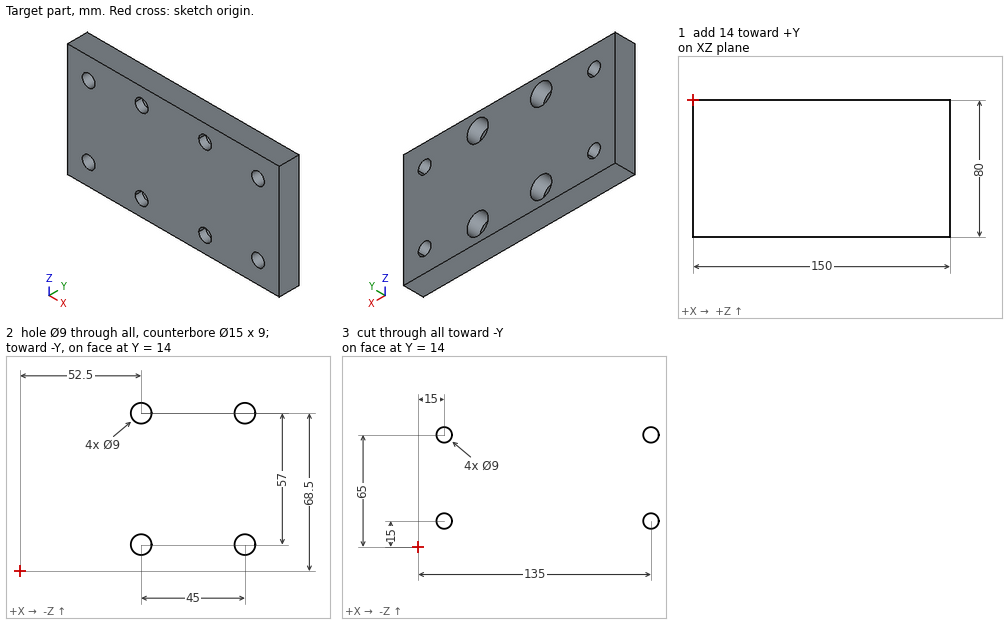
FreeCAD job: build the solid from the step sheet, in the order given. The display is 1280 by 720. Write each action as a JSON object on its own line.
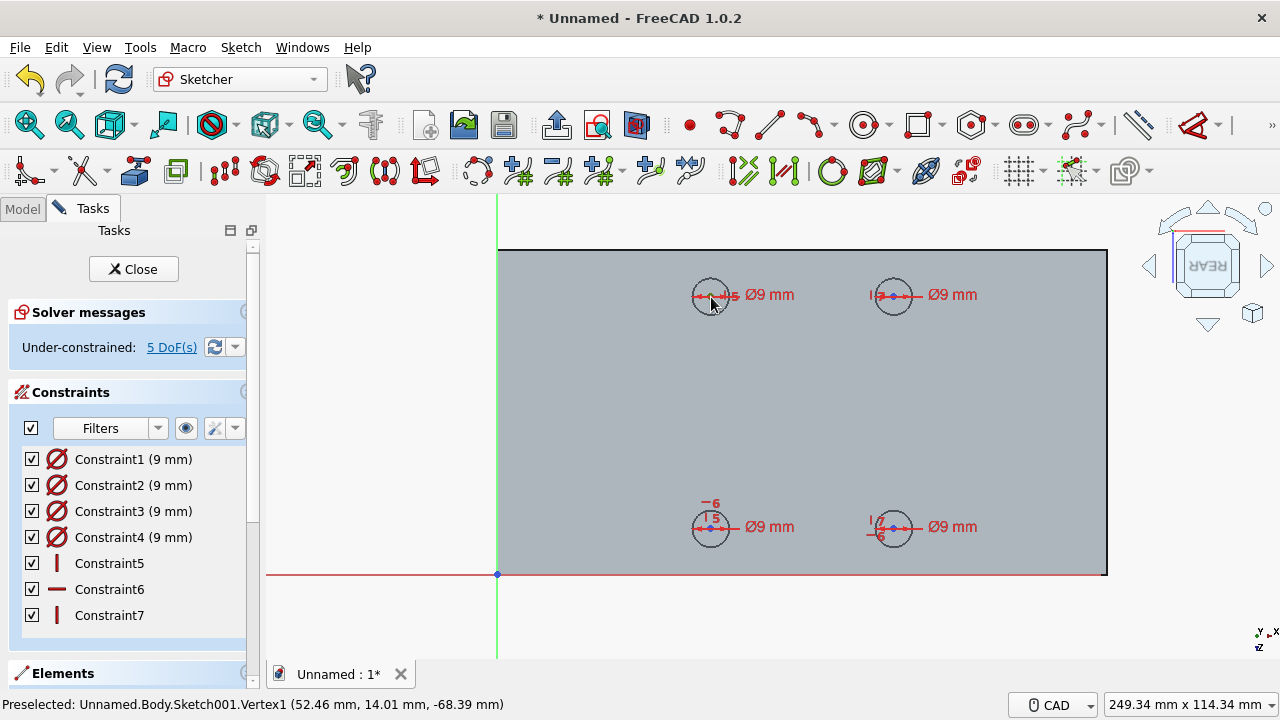
{"action": "left_click", "coordinate": [894, 297]}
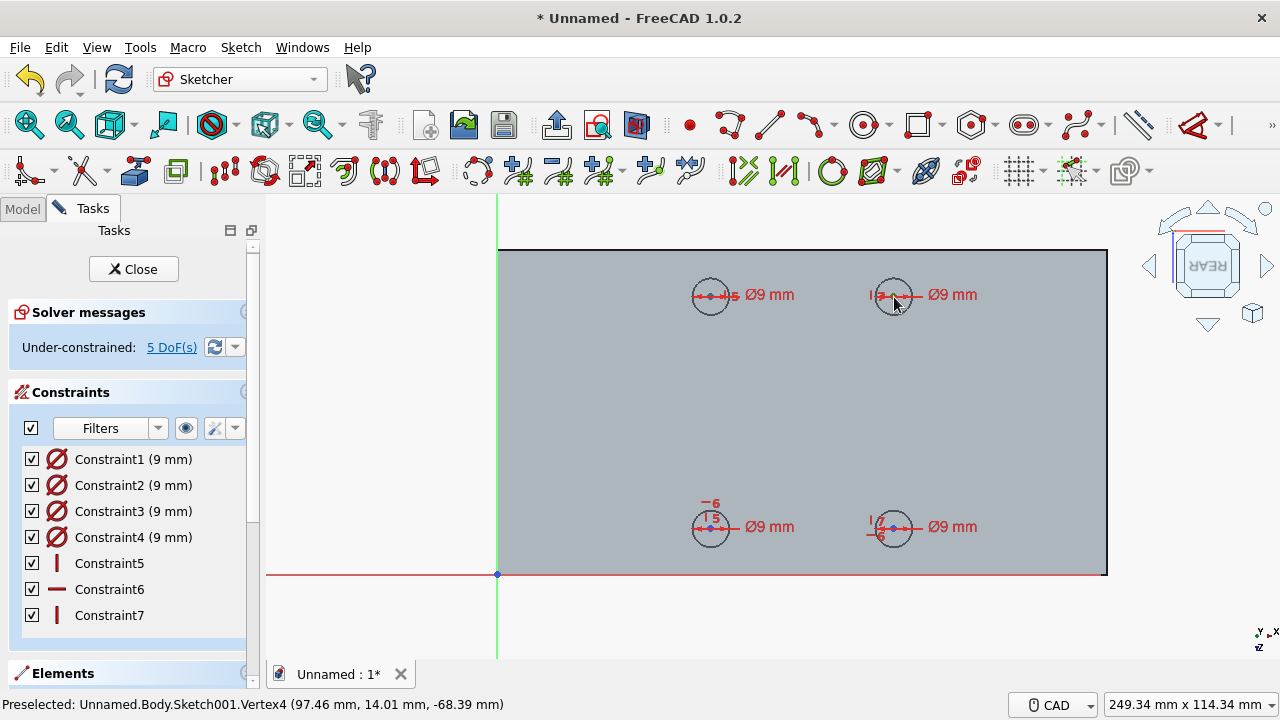
{"action": "key", "text": "h"}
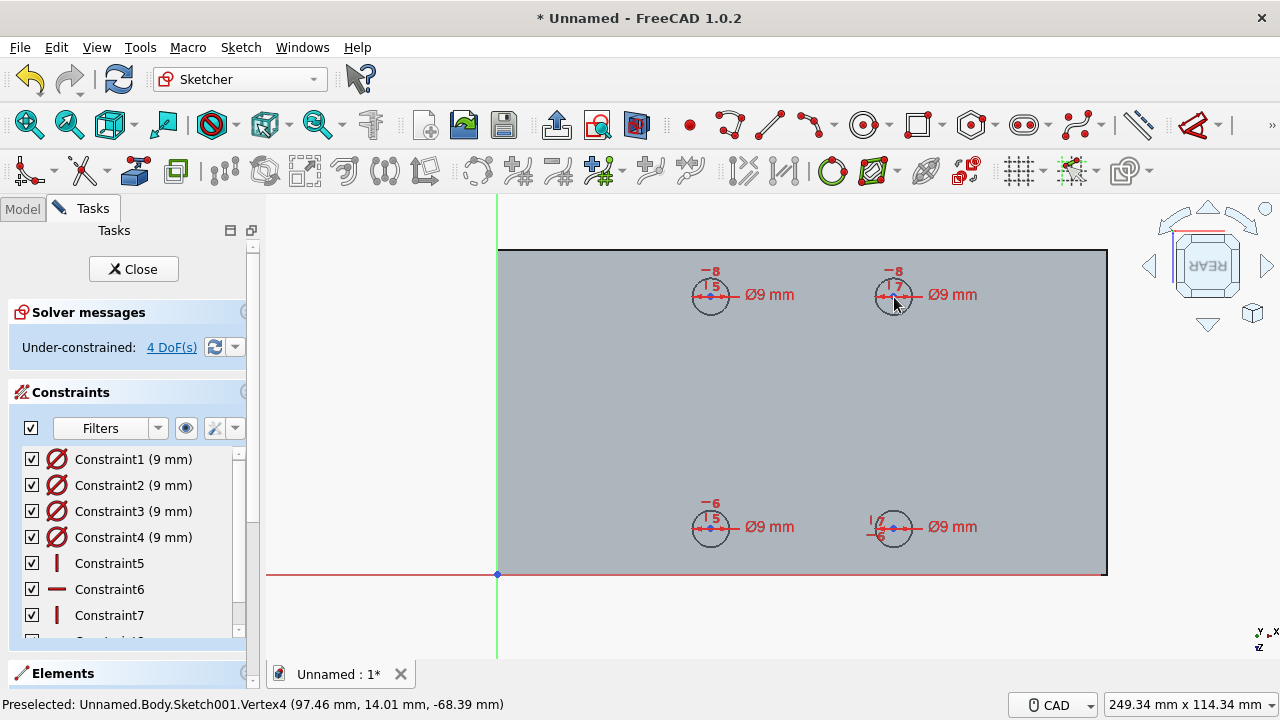
{"action": "left_click", "coordinate": [711, 297]}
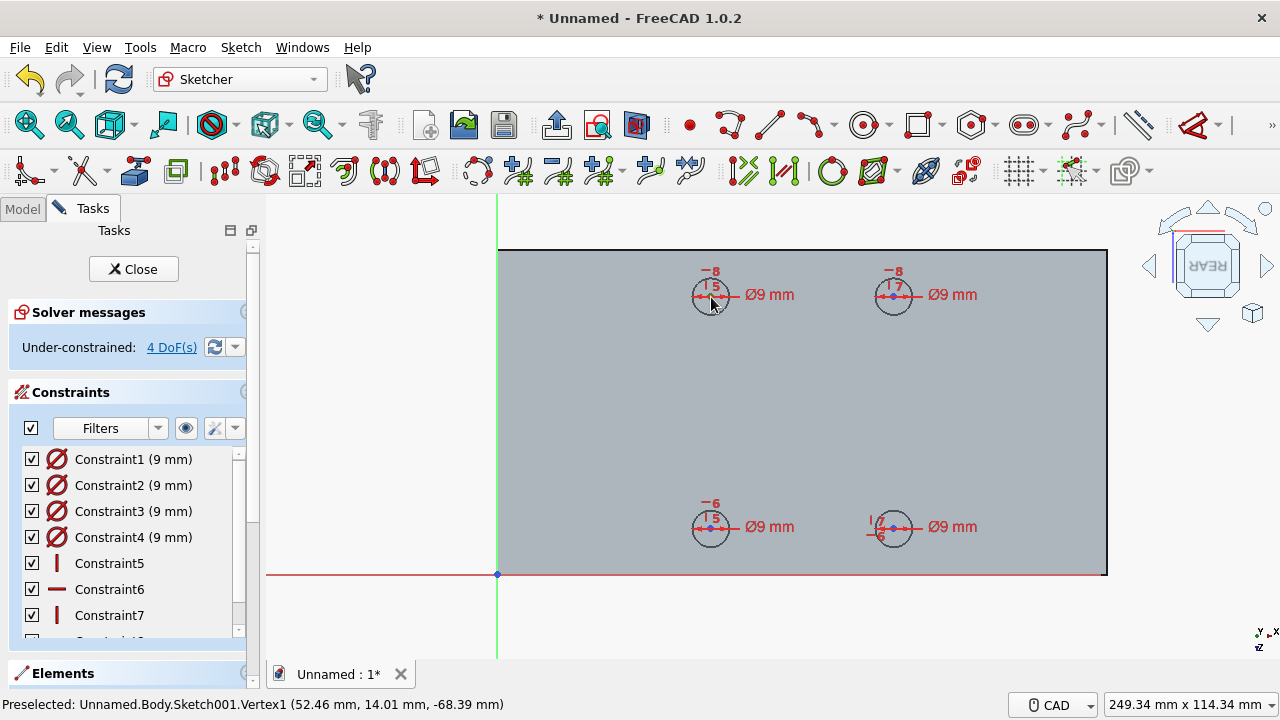
{"action": "left_click", "coordinate": [711, 529]}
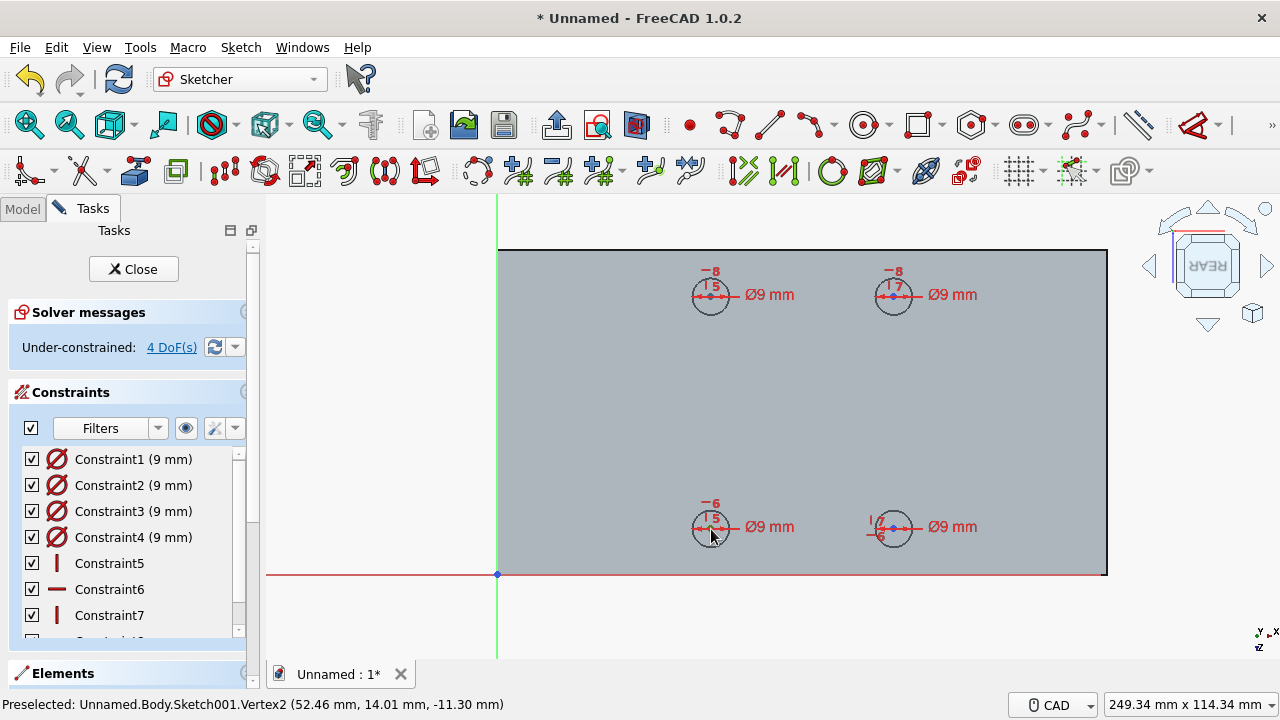
{"action": "left_click", "coordinate": [1220, 126]}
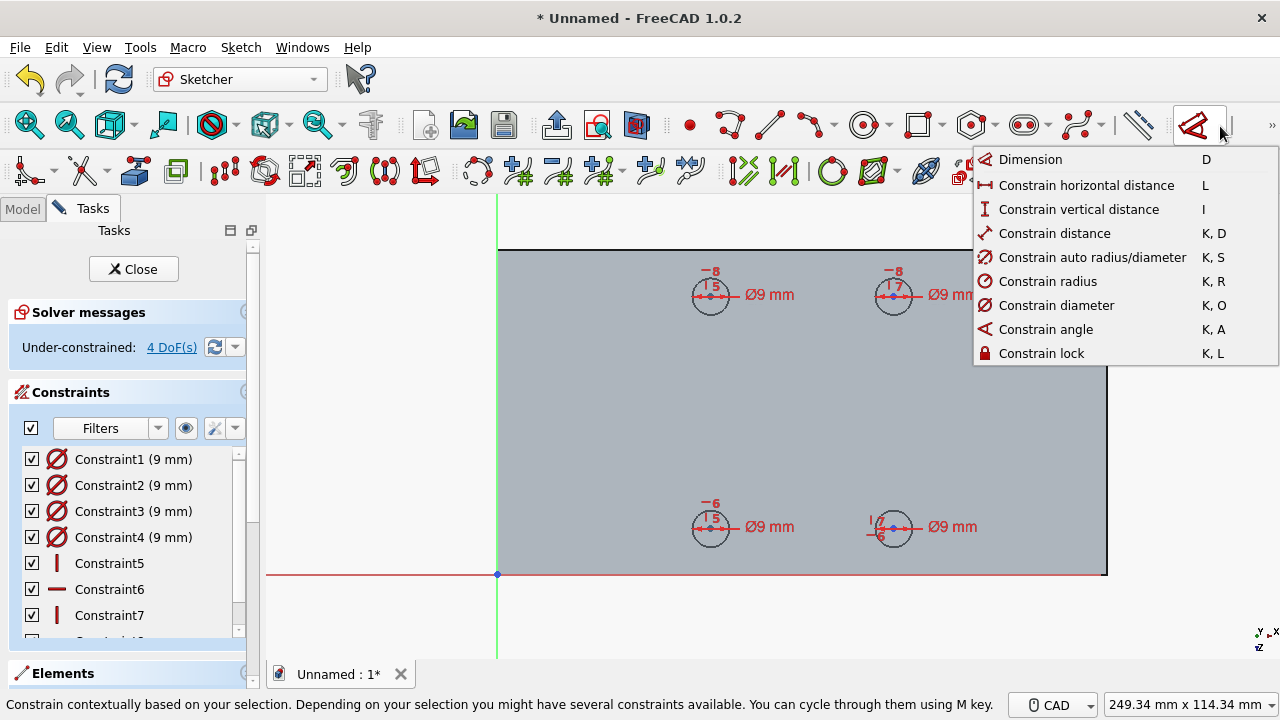
{"action": "left_click", "coordinate": [1126, 209]}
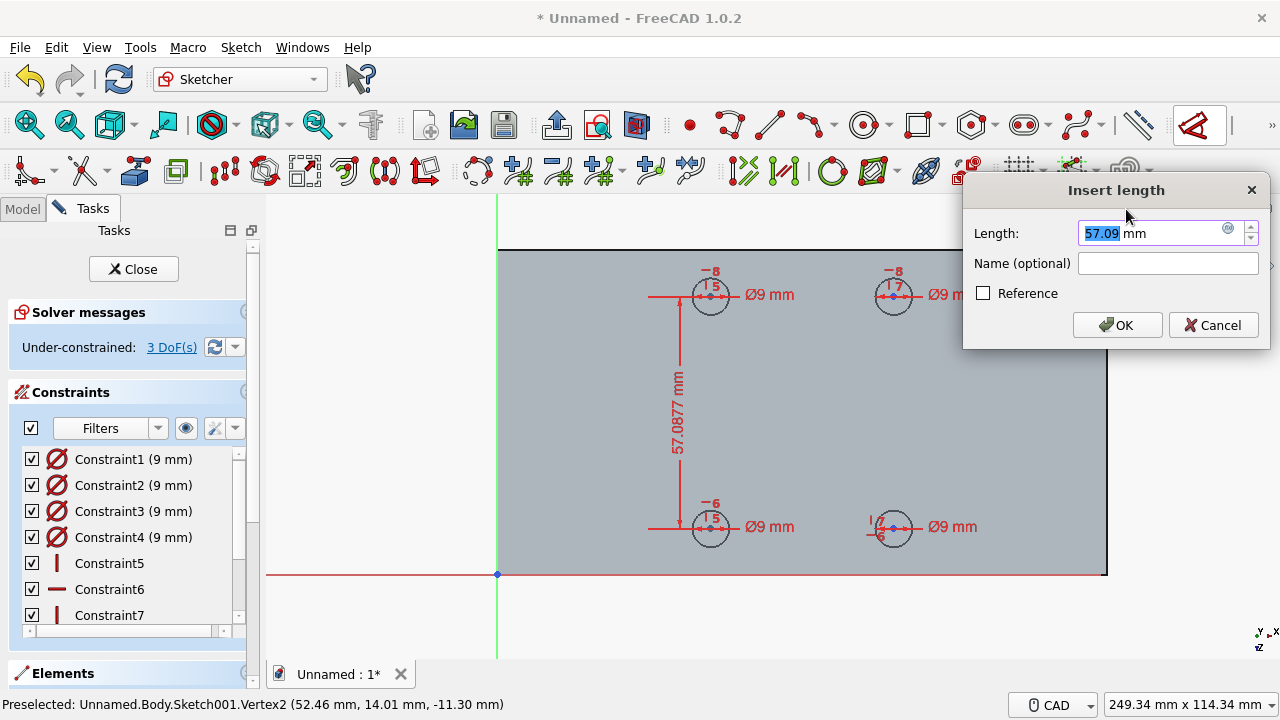
{"action": "type", "text": "57"}
{"action": "key", "text": "Return"}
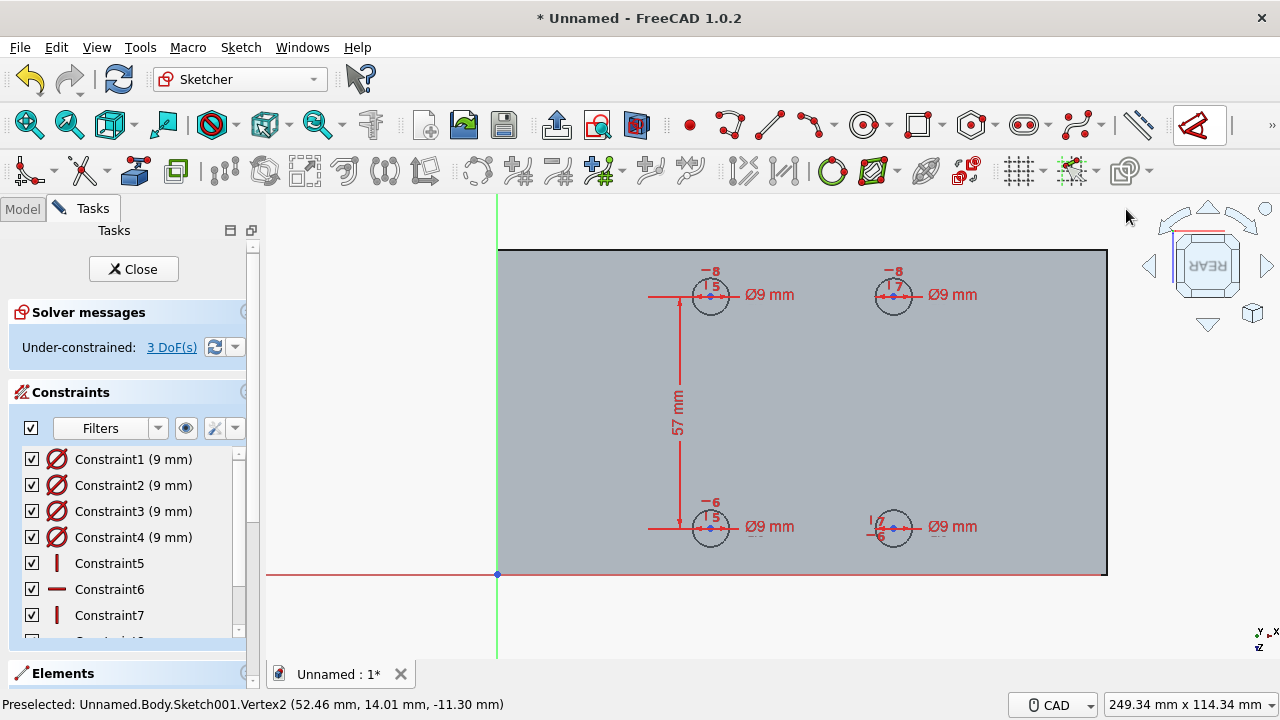
{"action": "left_click", "coordinate": [711, 529]}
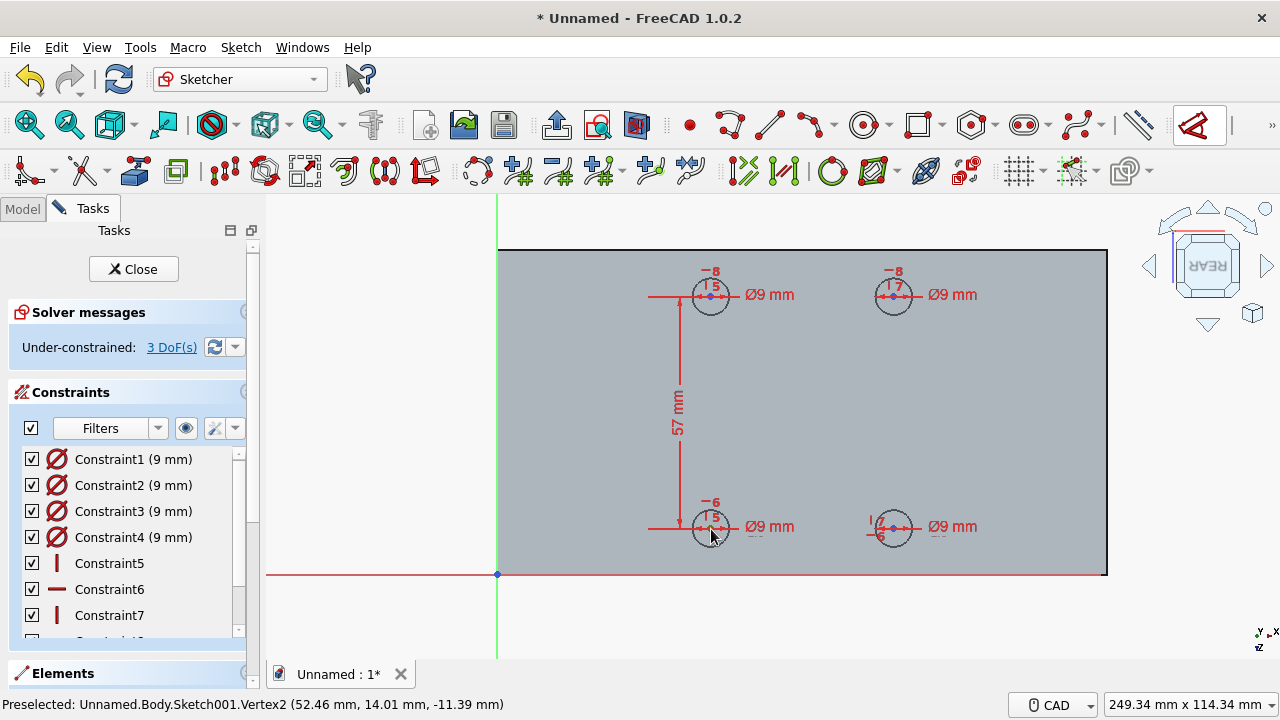
{"action": "left_click", "coordinate": [894, 529]}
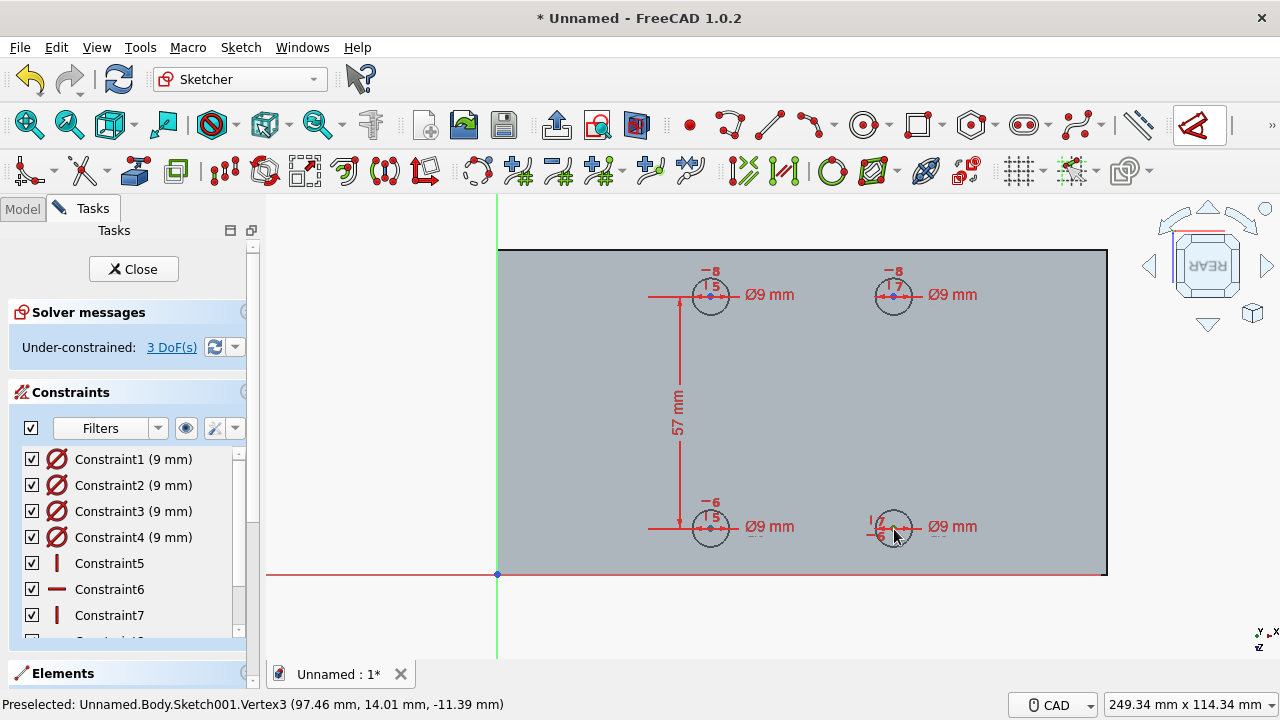
{"action": "key", "text": "l"}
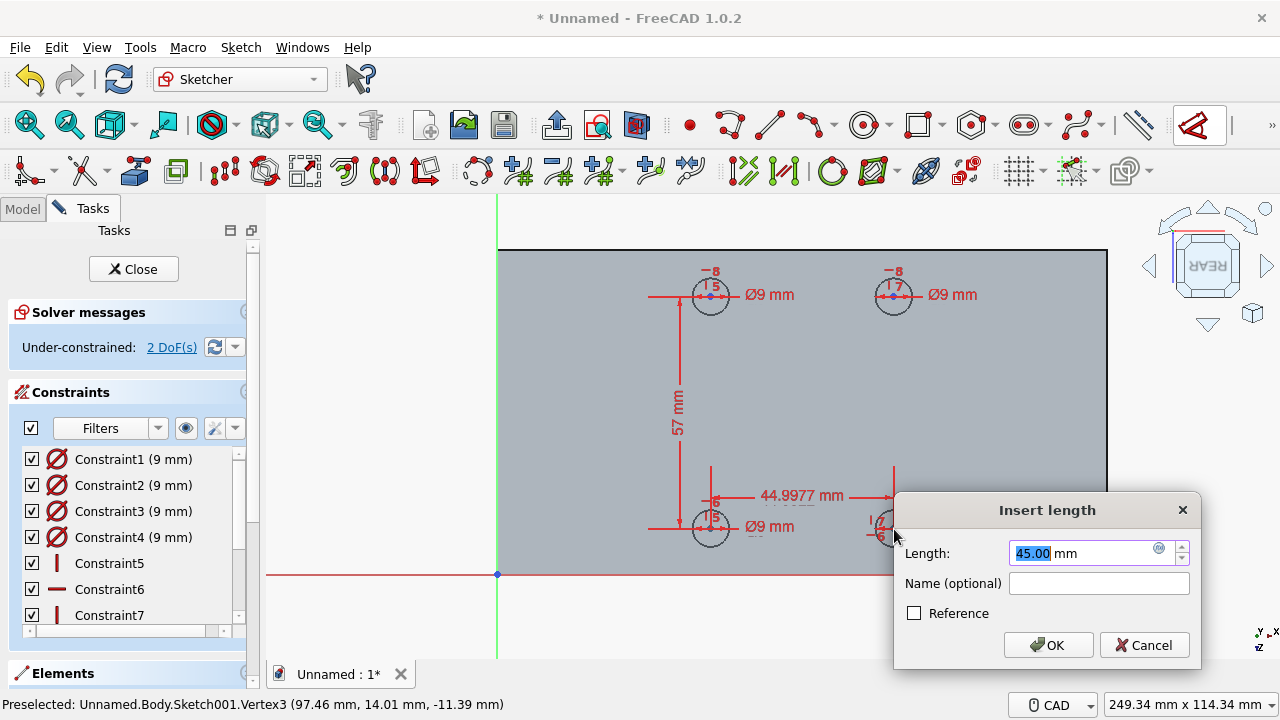
{"action": "type", "text": "45"}
{"action": "key", "text": "Return"}